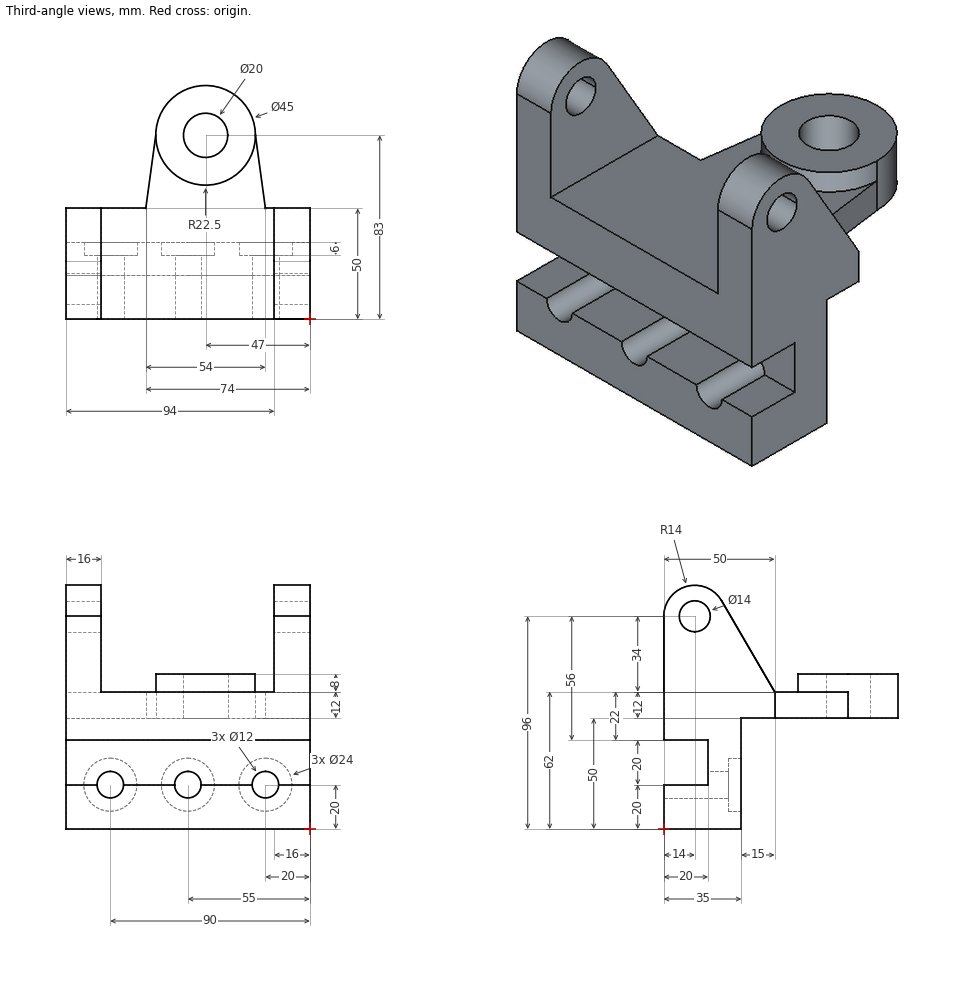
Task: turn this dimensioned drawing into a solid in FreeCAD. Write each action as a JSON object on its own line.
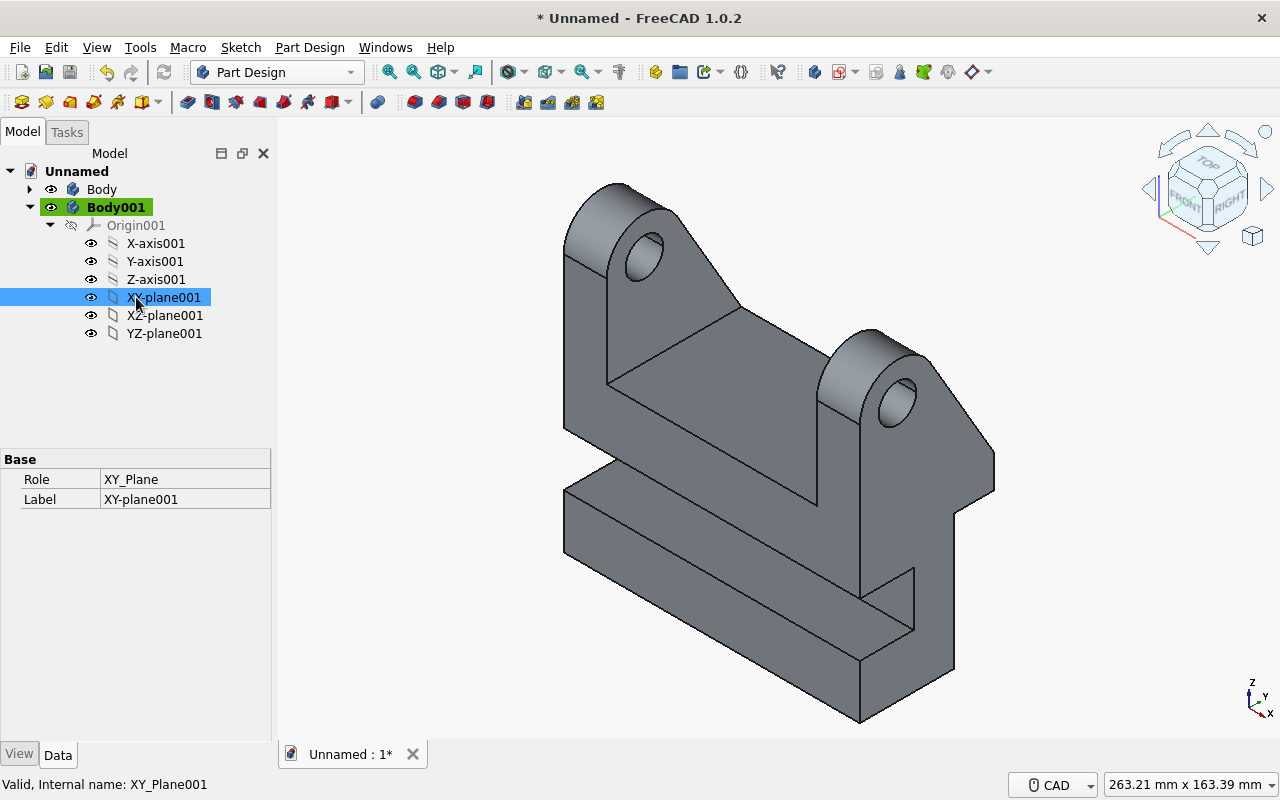
{"action": "left_click", "coordinate": [972, 72]}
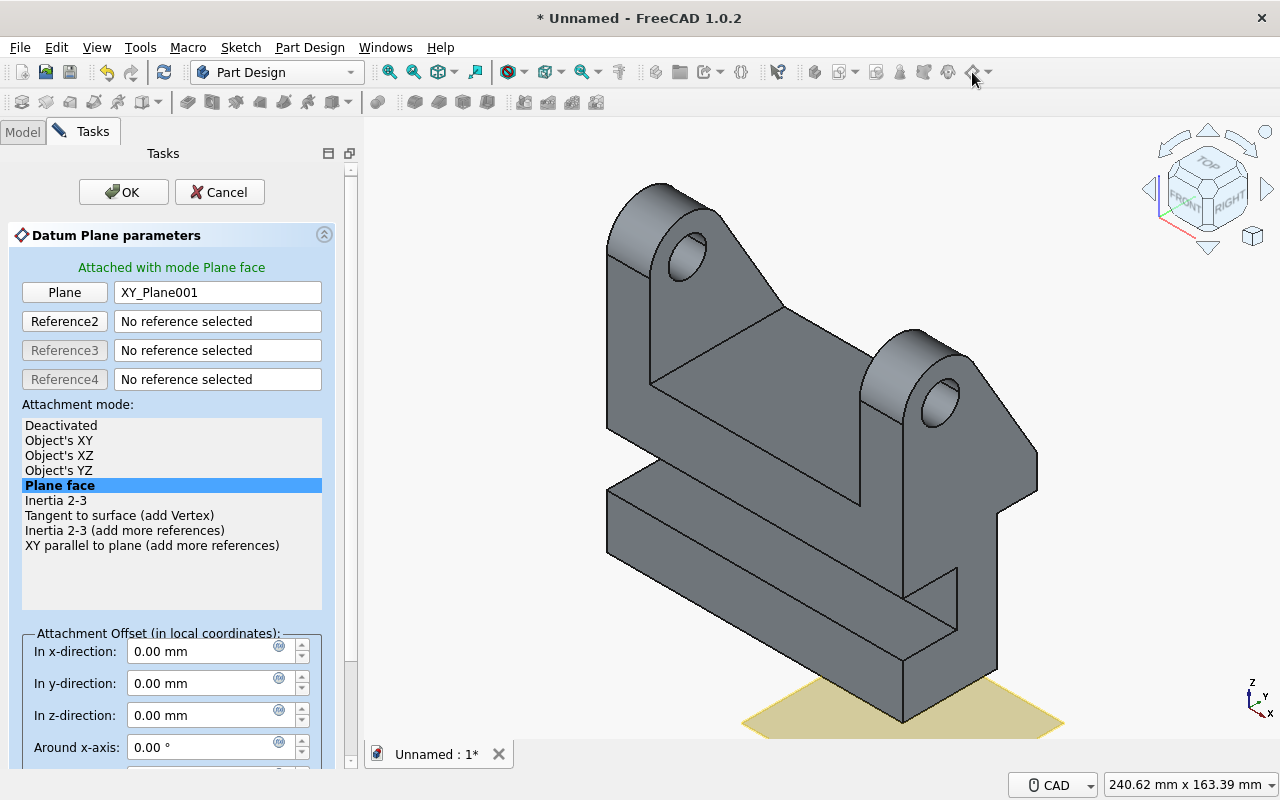
{"action": "triple_click", "coordinate": [210, 715]}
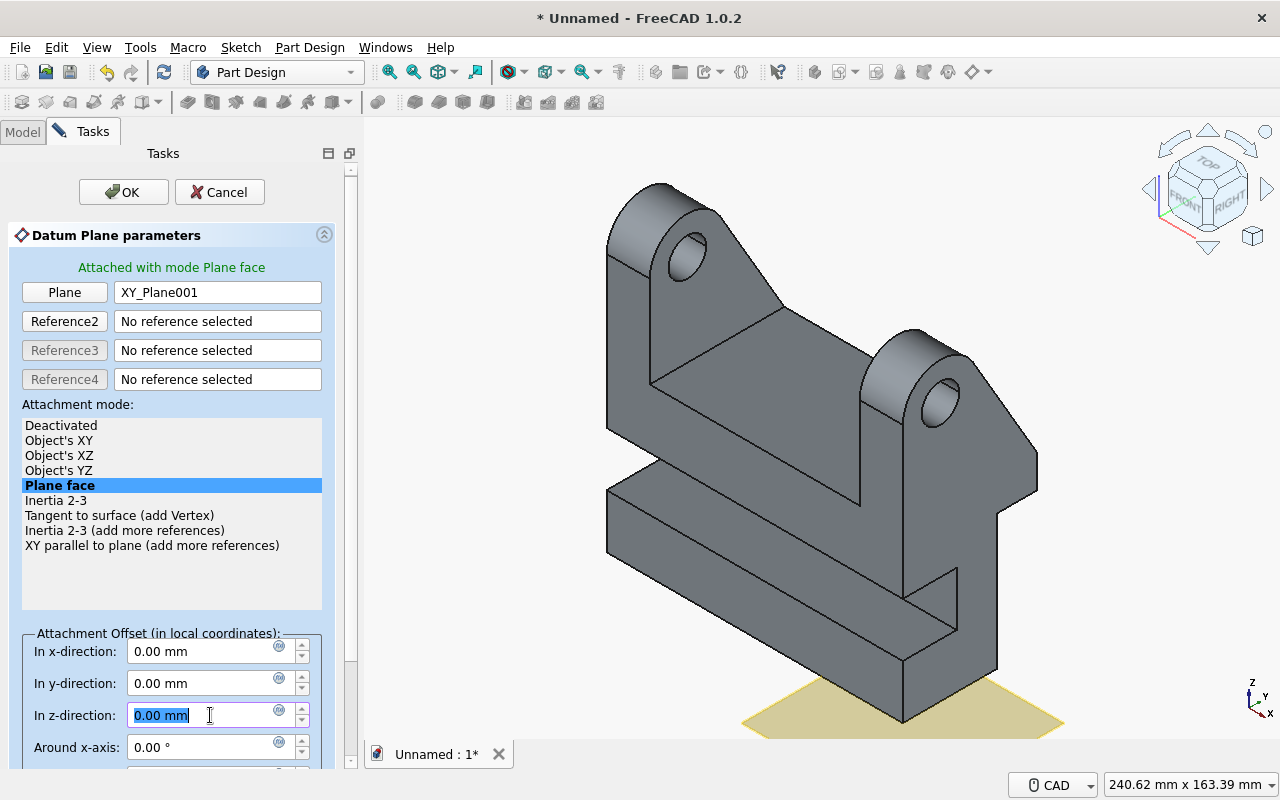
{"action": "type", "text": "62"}
{"action": "key", "text": "Tab"}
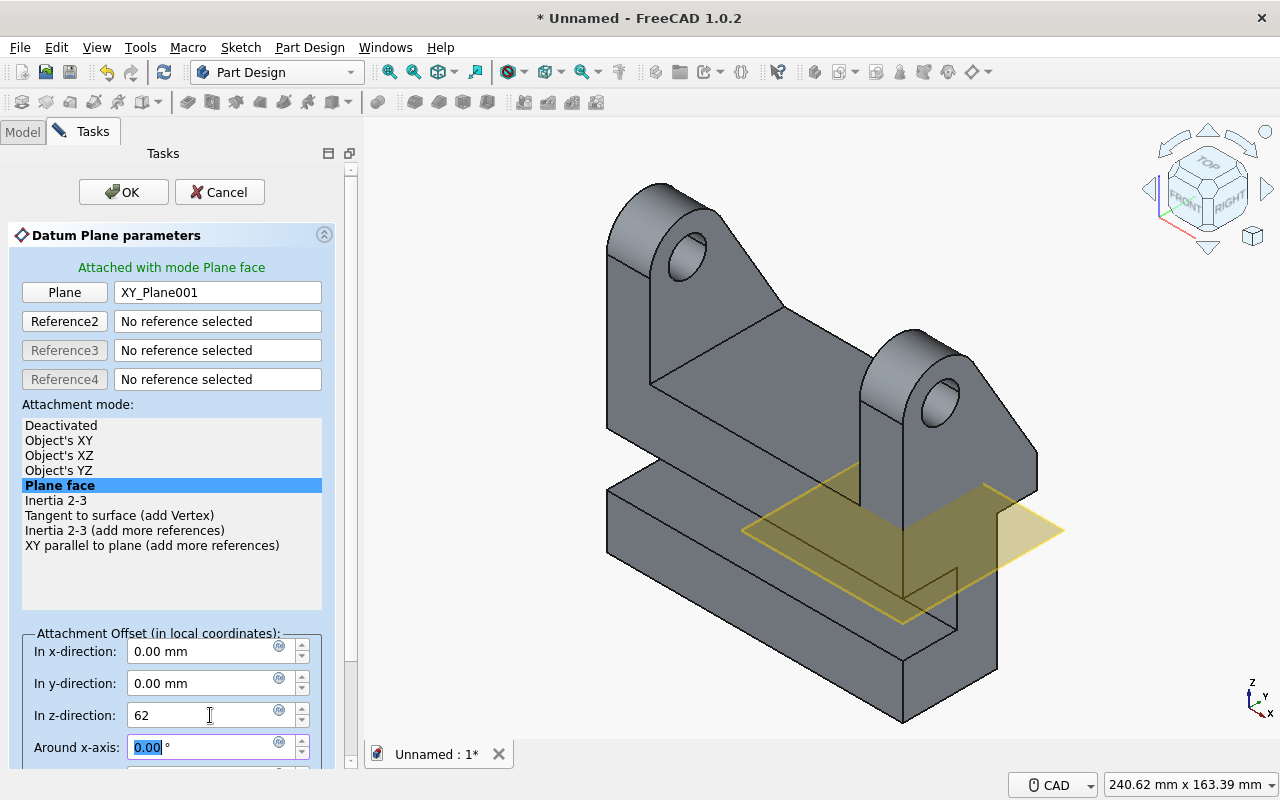
{"action": "left_click", "coordinate": [124, 192]}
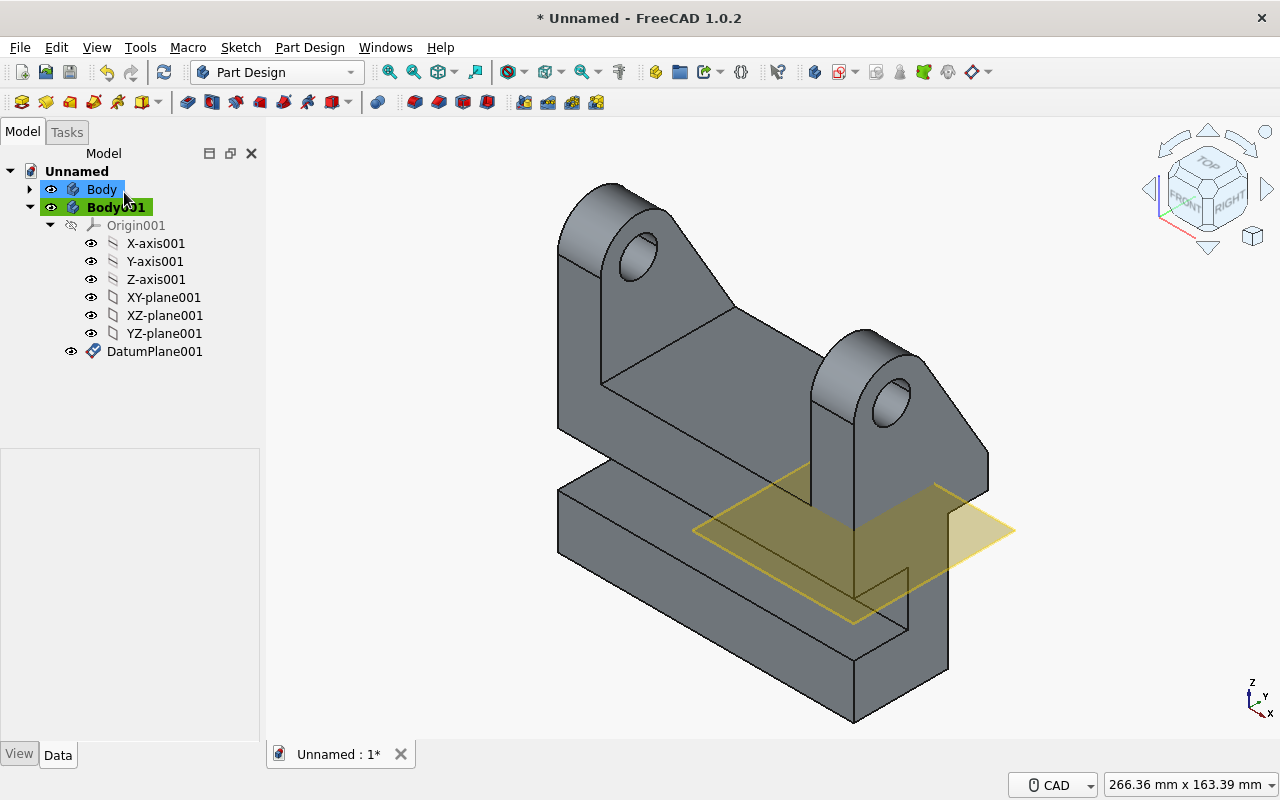
{"action": "left_click", "coordinate": [116, 351]}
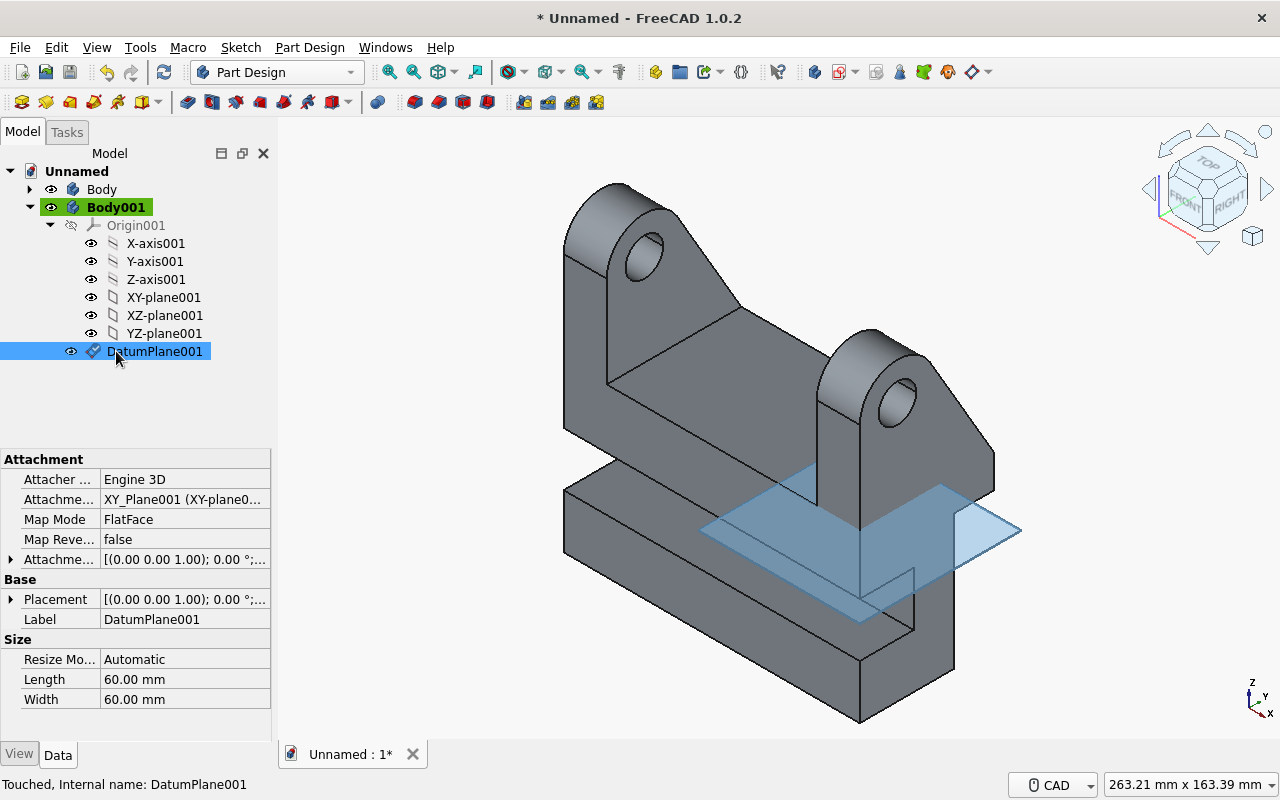
{"action": "left_click", "coordinate": [840, 72]}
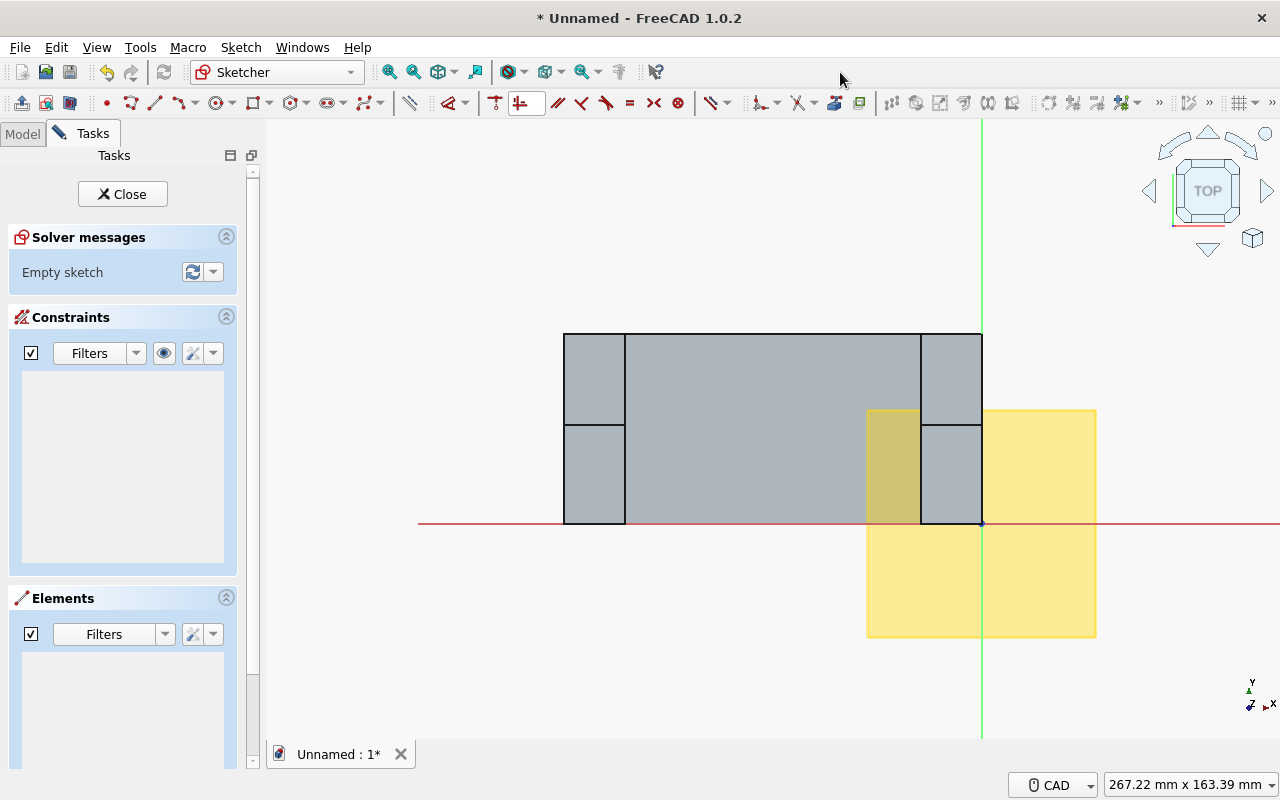
{"action": "scroll", "coordinate": [294, 711], "scroll_direction": "down", "scroll_amount": 1}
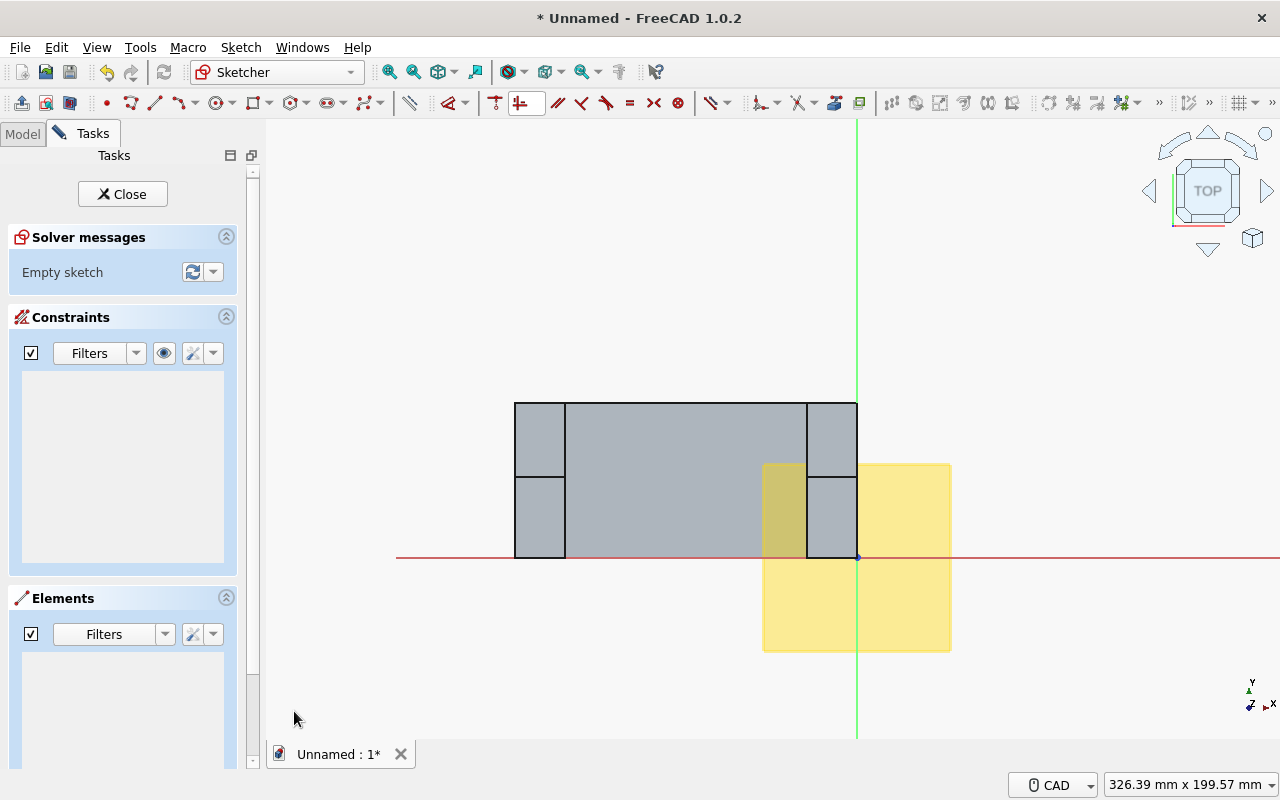
{"action": "left_click", "coordinate": [216, 104]}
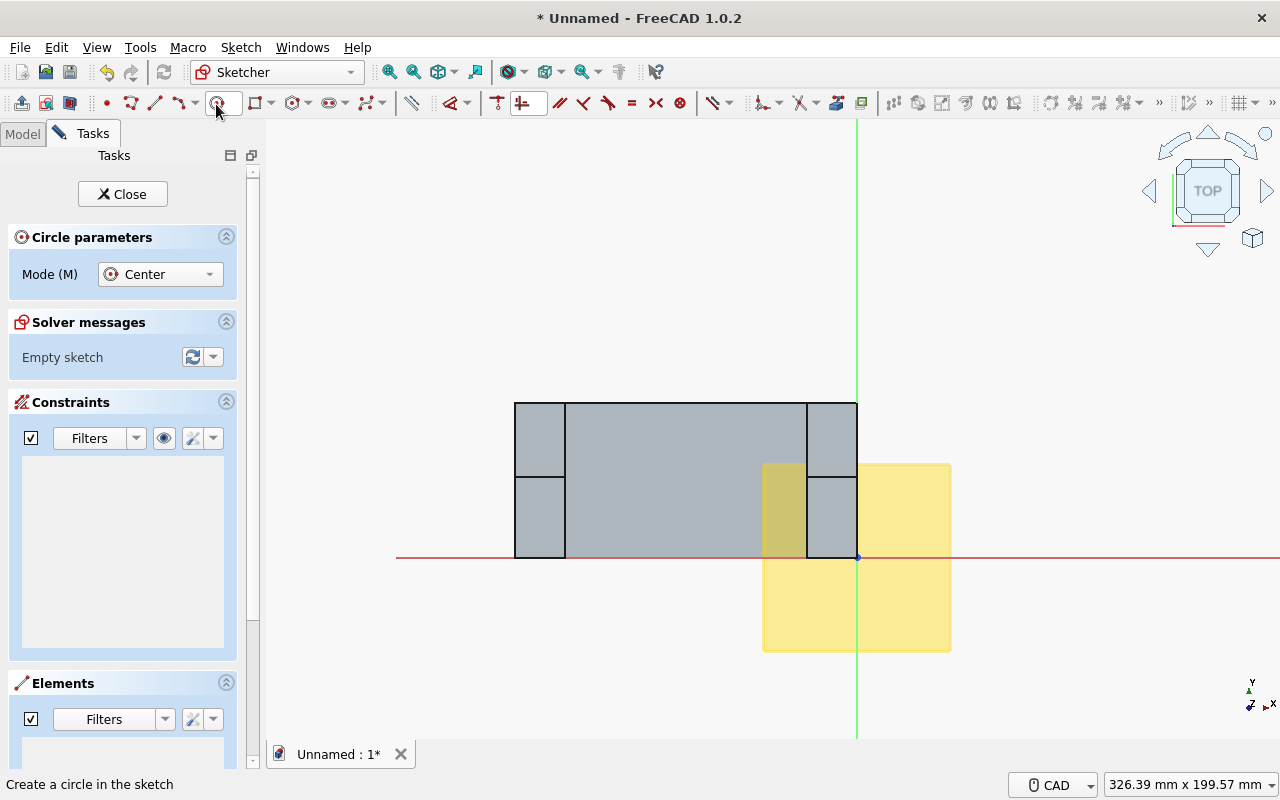
{"action": "left_click", "coordinate": [711, 300]}
{"action": "mouse_move", "coordinate": [760, 251]}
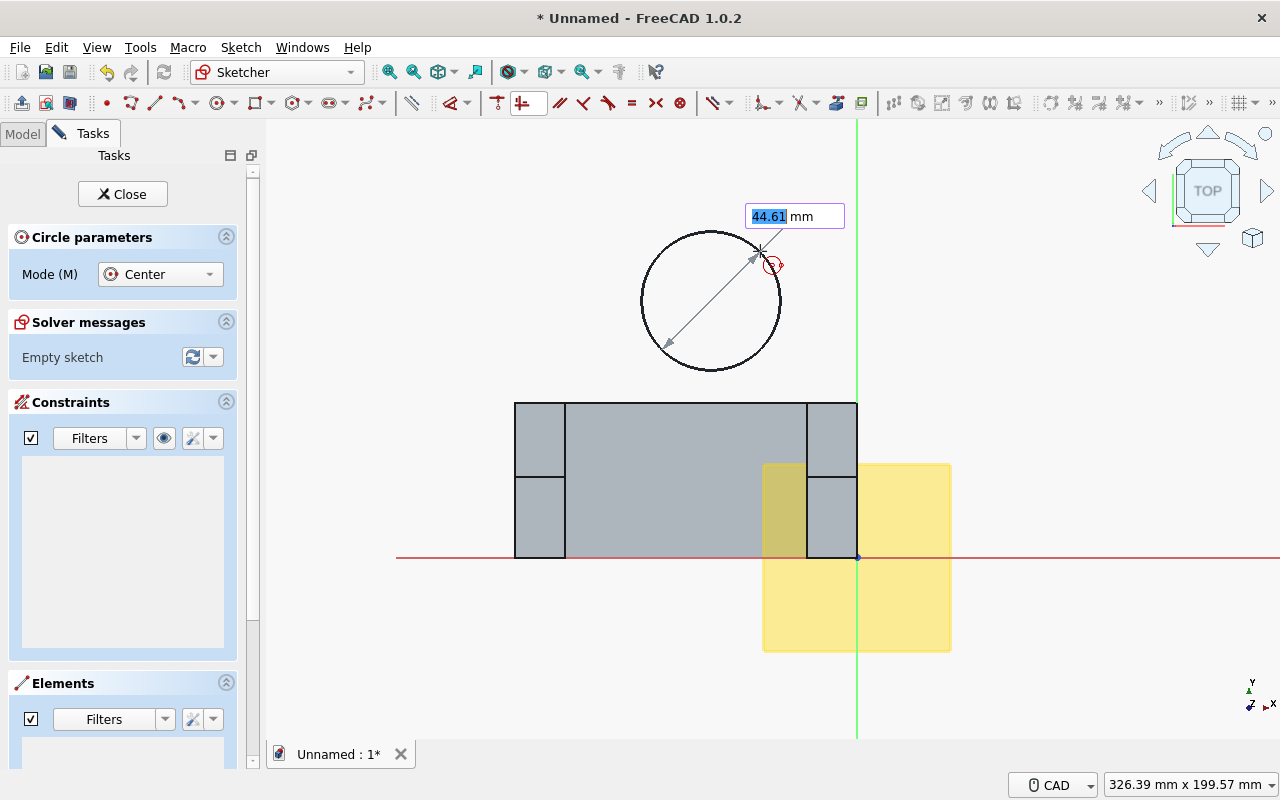
{"action": "type", "text": "45"}
{"action": "key", "text": "Return"}
{"action": "key", "text": "Escape"}